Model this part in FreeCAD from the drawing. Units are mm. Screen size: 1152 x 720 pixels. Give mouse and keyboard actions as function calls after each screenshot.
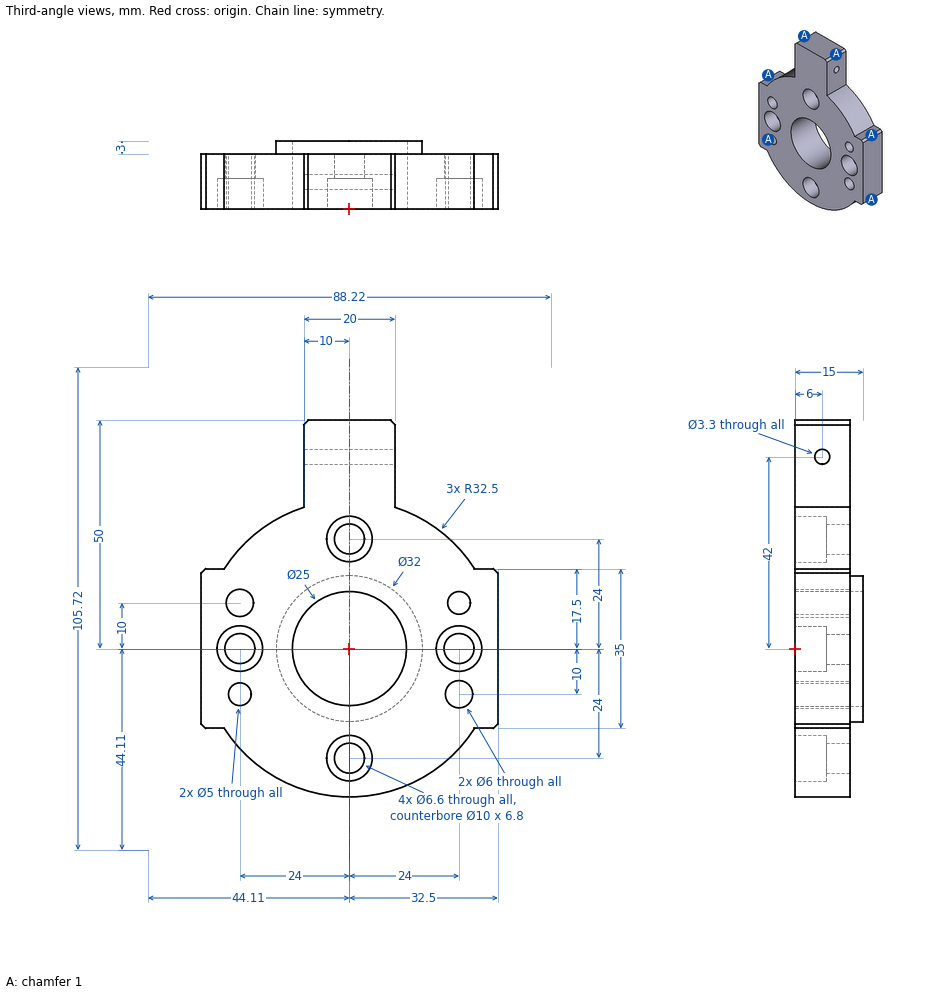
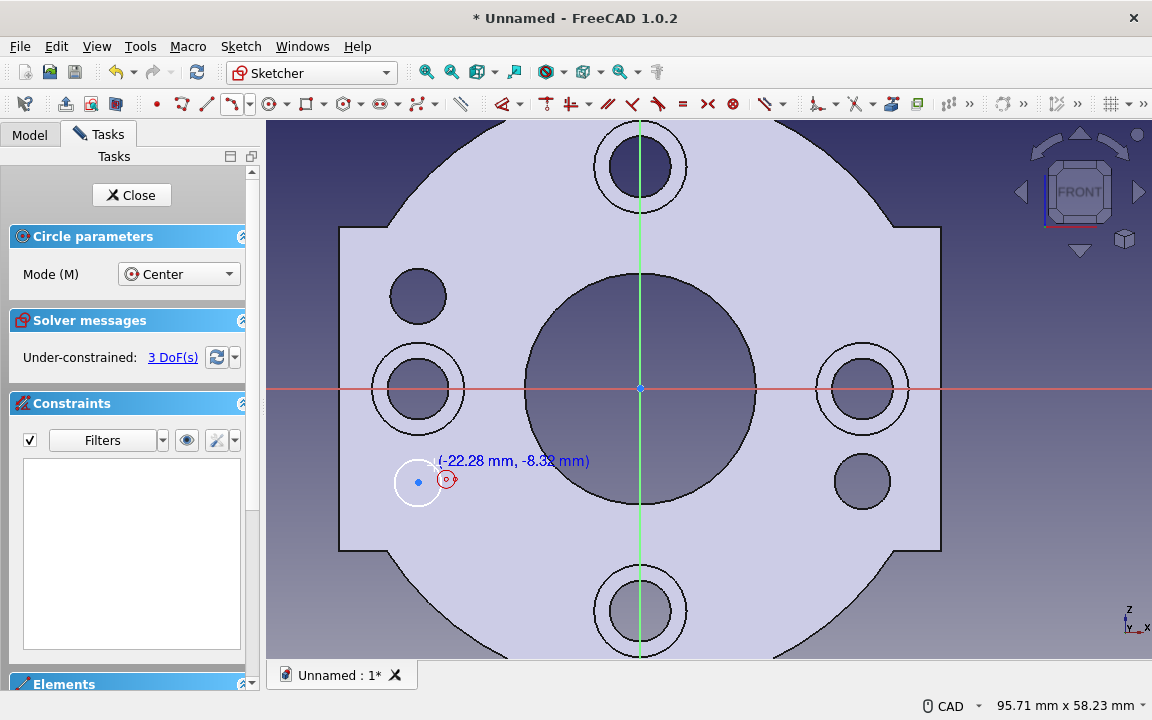
click(862, 296)
click(879, 280)
key(Escape)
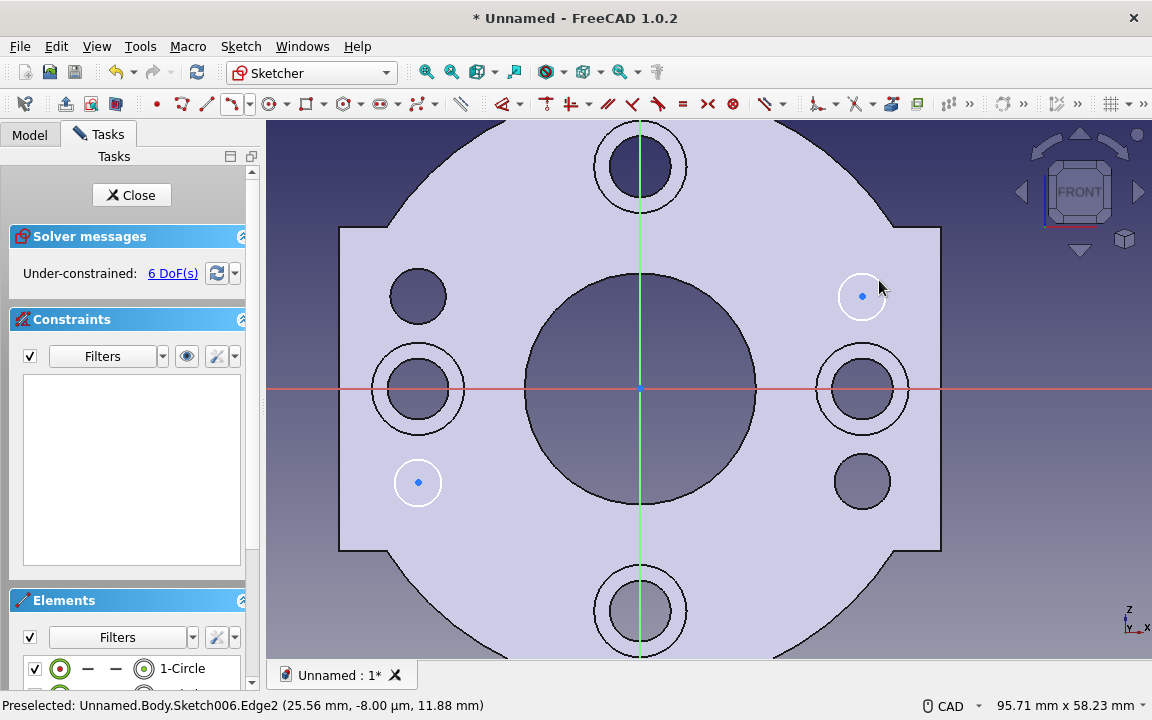
click(434, 466)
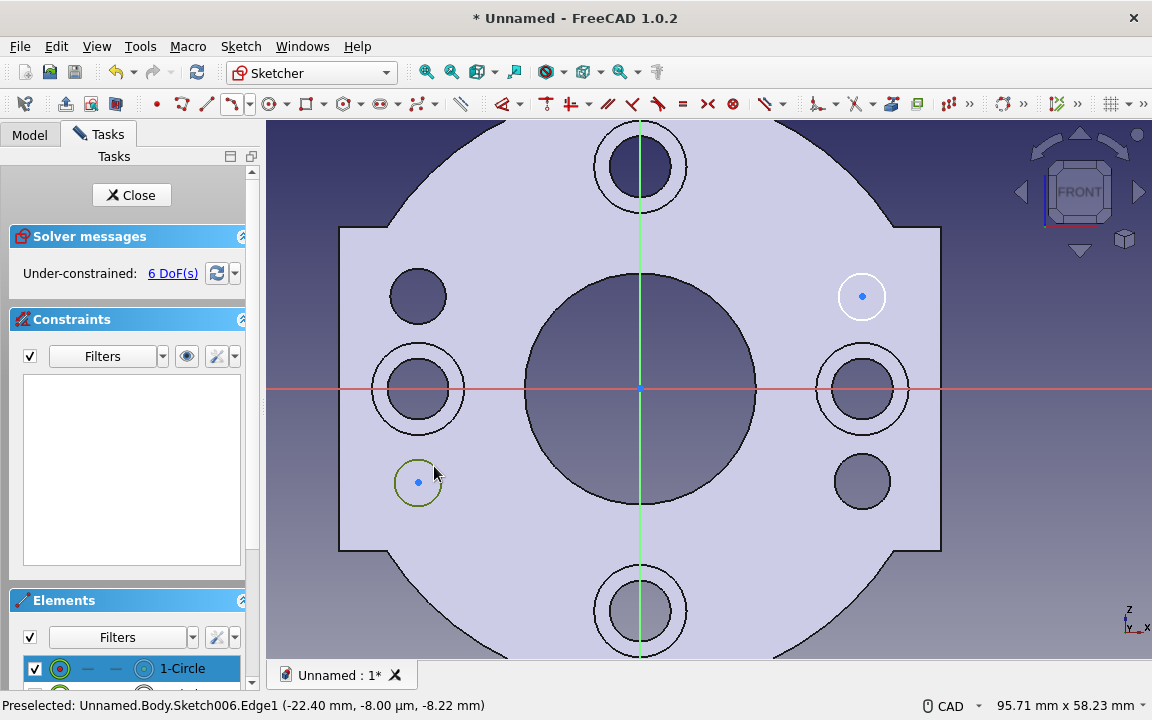
click(878, 280)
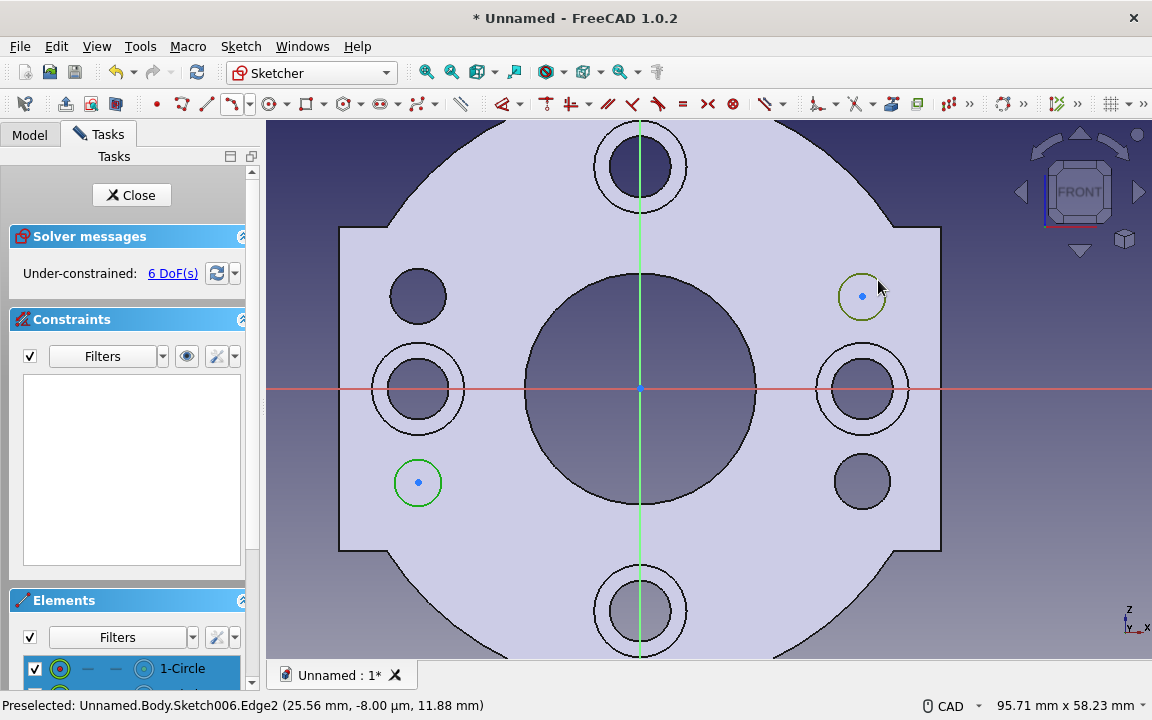
click(683, 104)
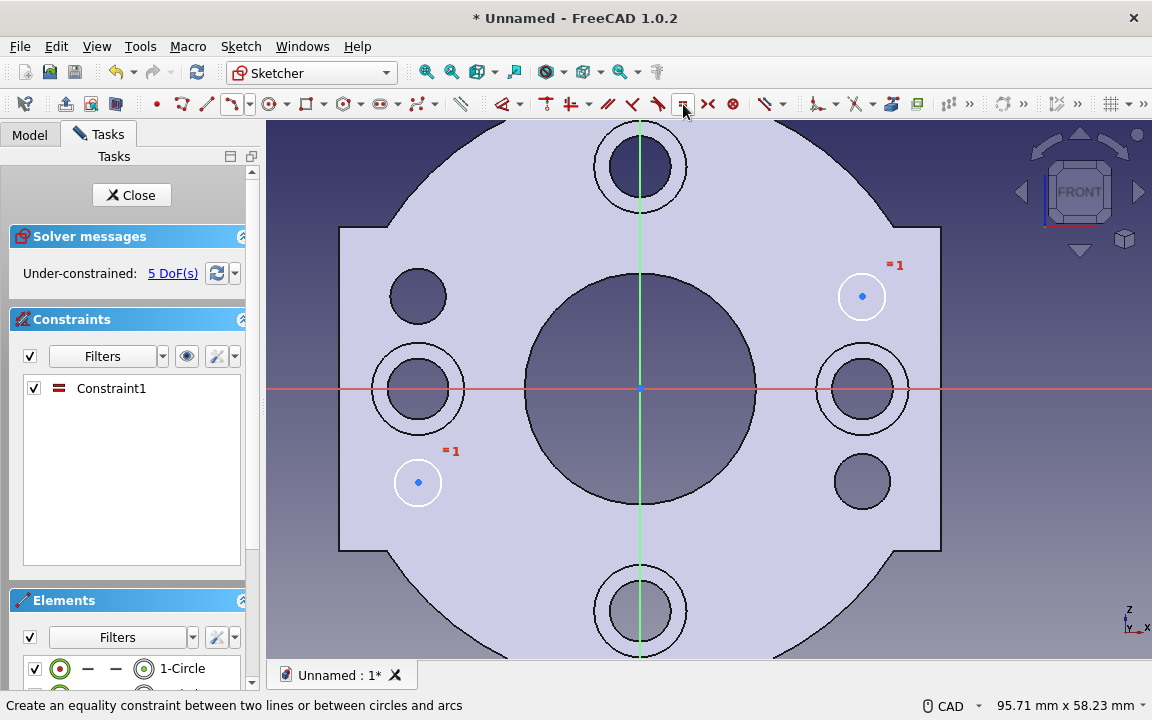
click(502, 104)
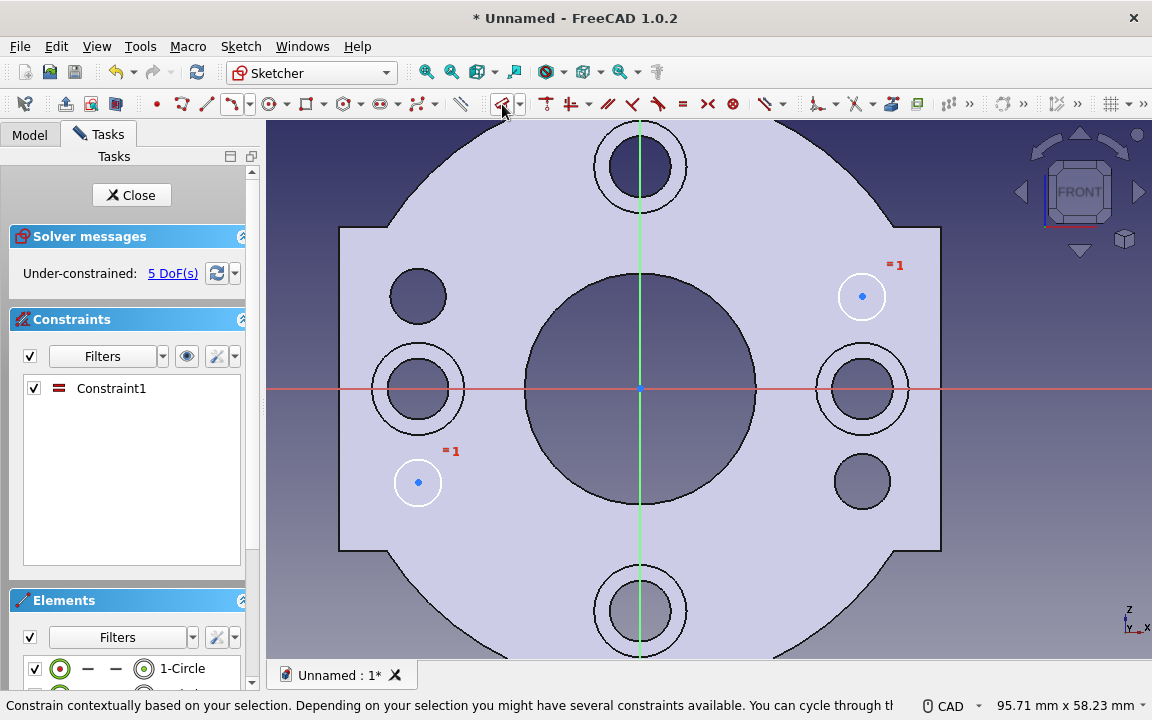
click(434, 466)
click(456, 443)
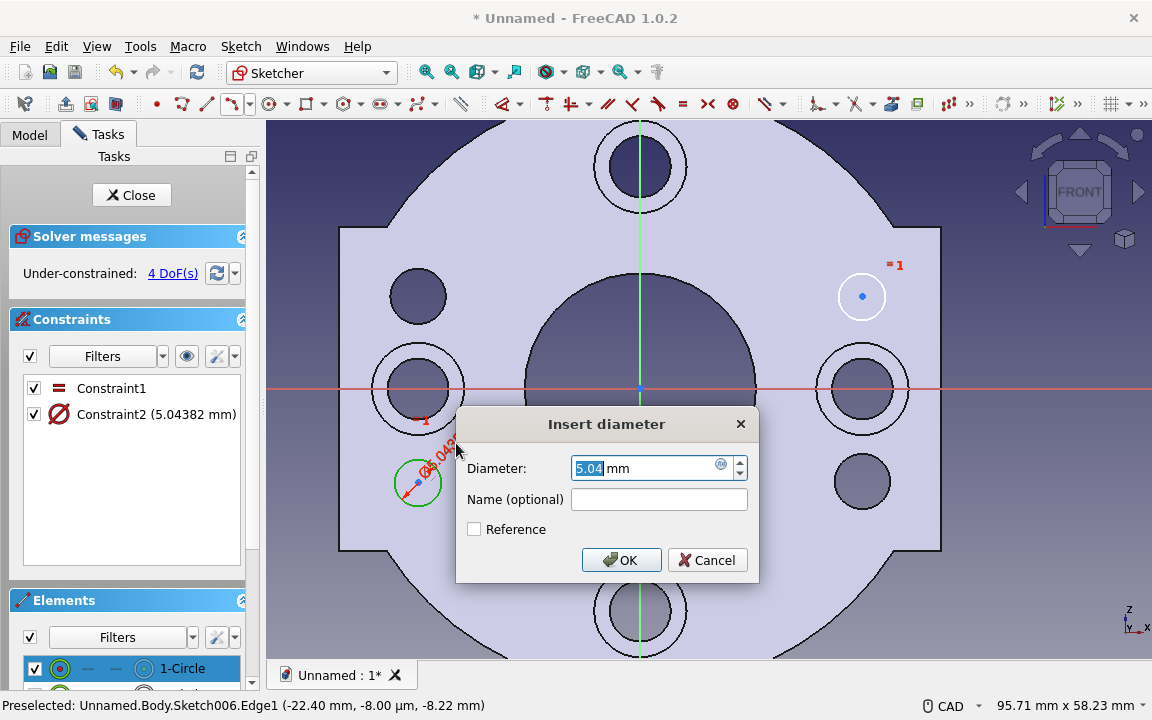
text(5)
key(Return)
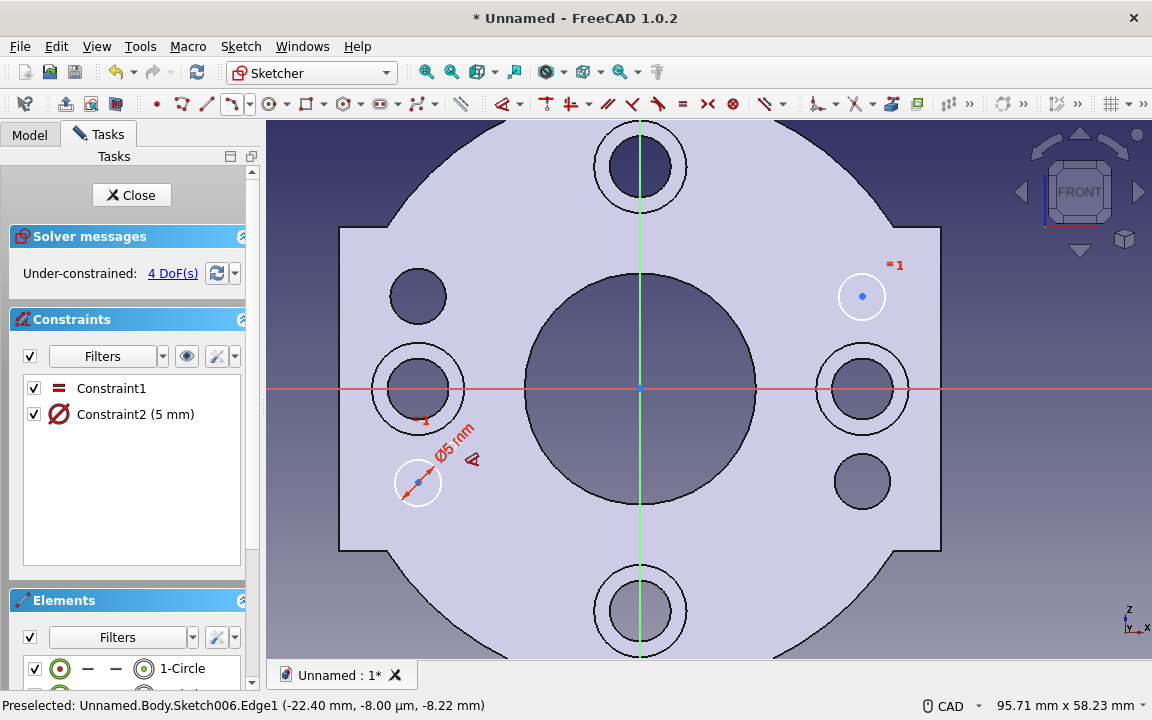
click(418, 483)
click(529, 517)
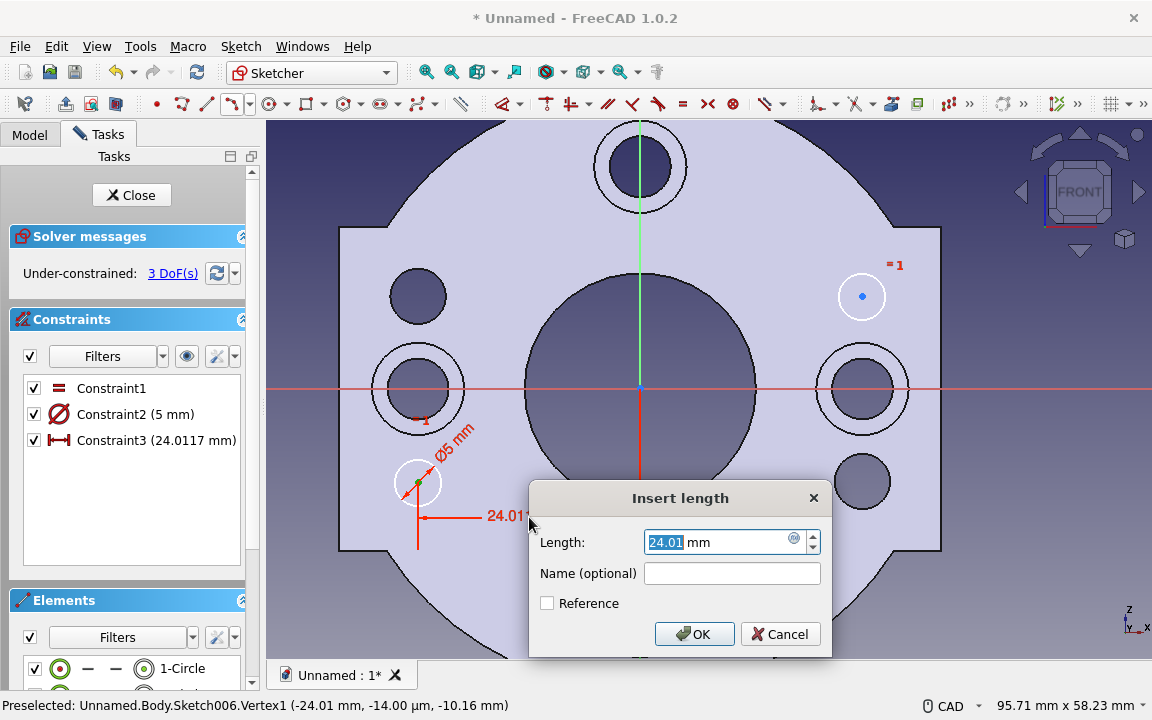
text(24)
key(Return)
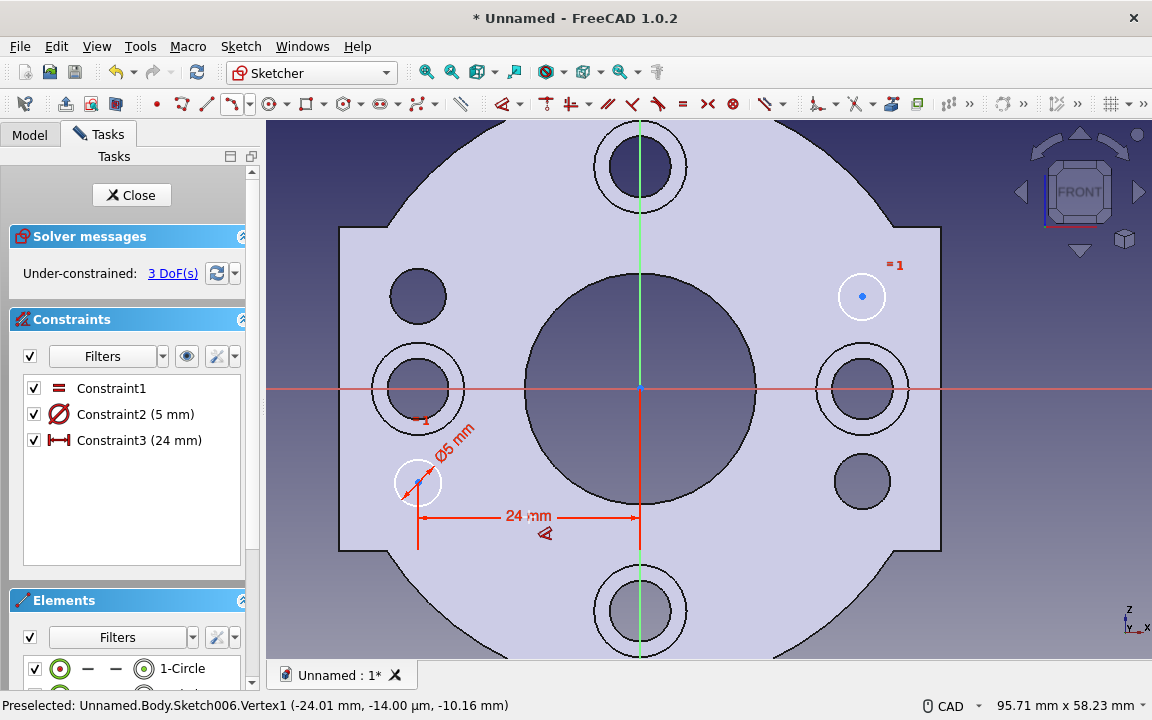
click(418, 483)
click(384, 436)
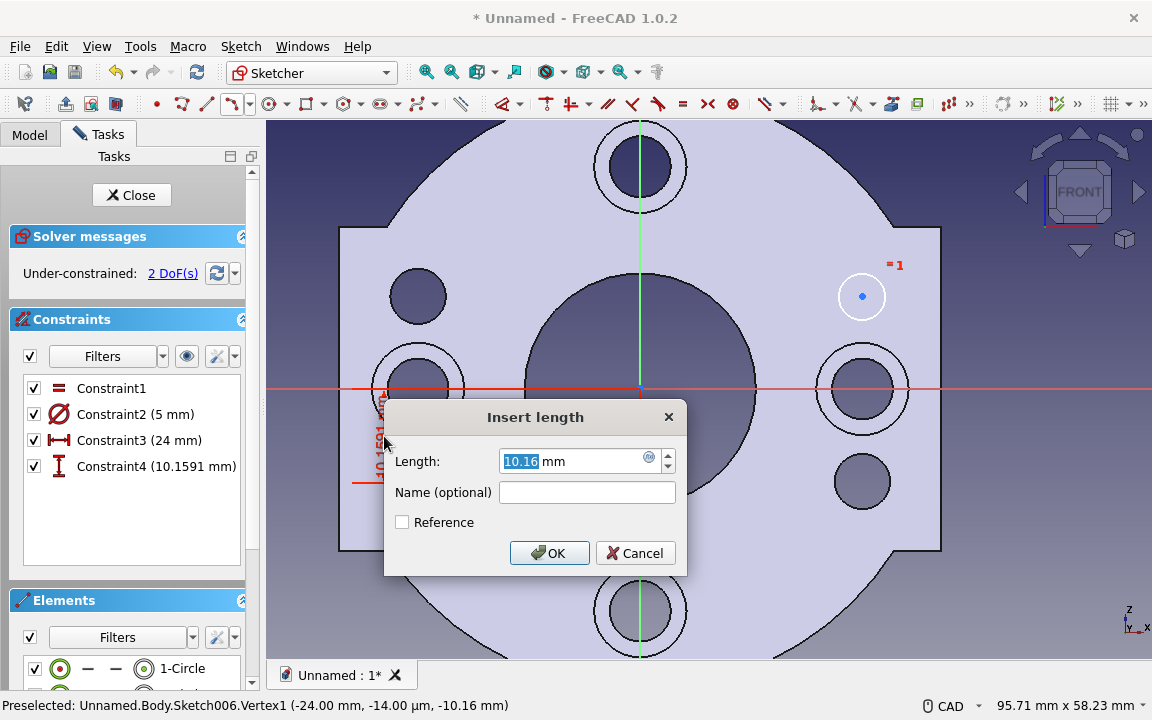
text(10)
key(Return)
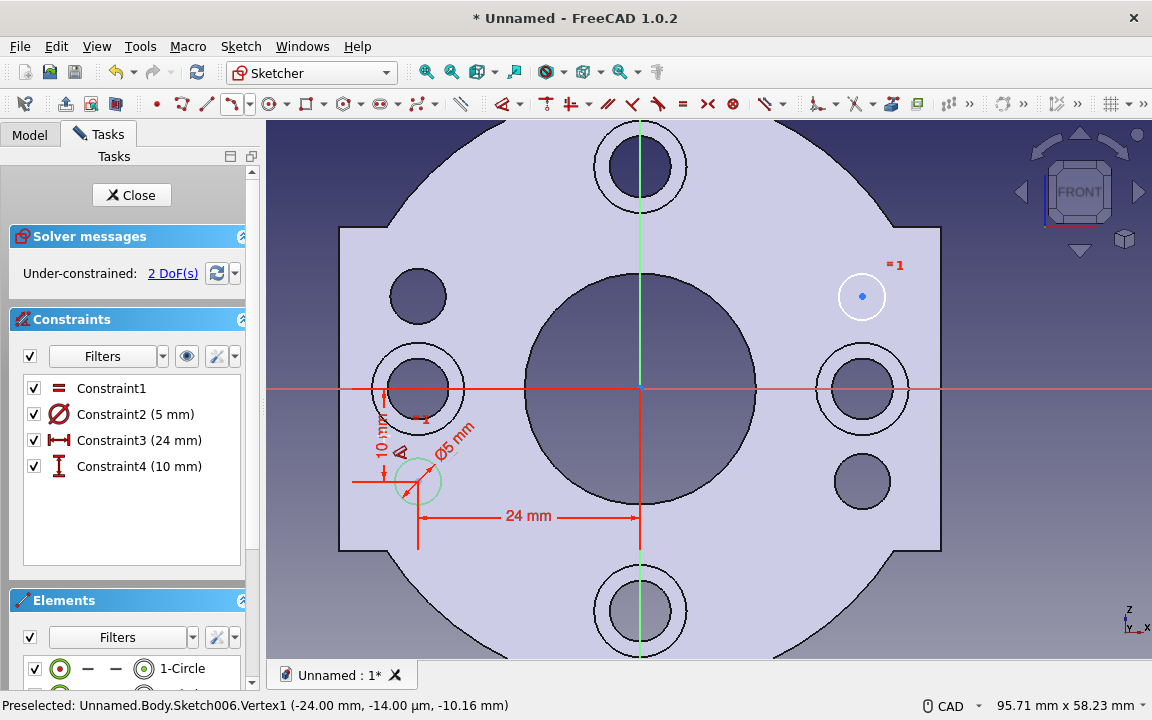
click(862, 297)
click(751, 263)